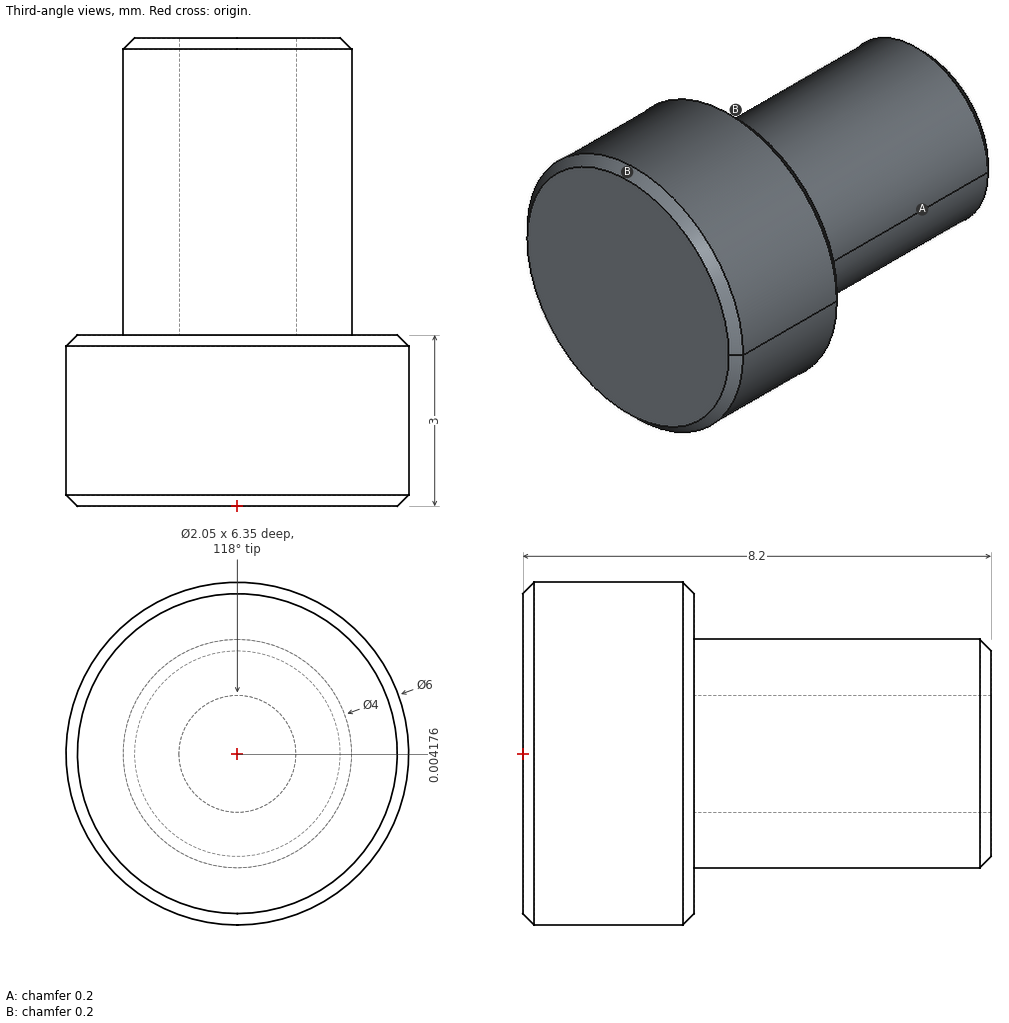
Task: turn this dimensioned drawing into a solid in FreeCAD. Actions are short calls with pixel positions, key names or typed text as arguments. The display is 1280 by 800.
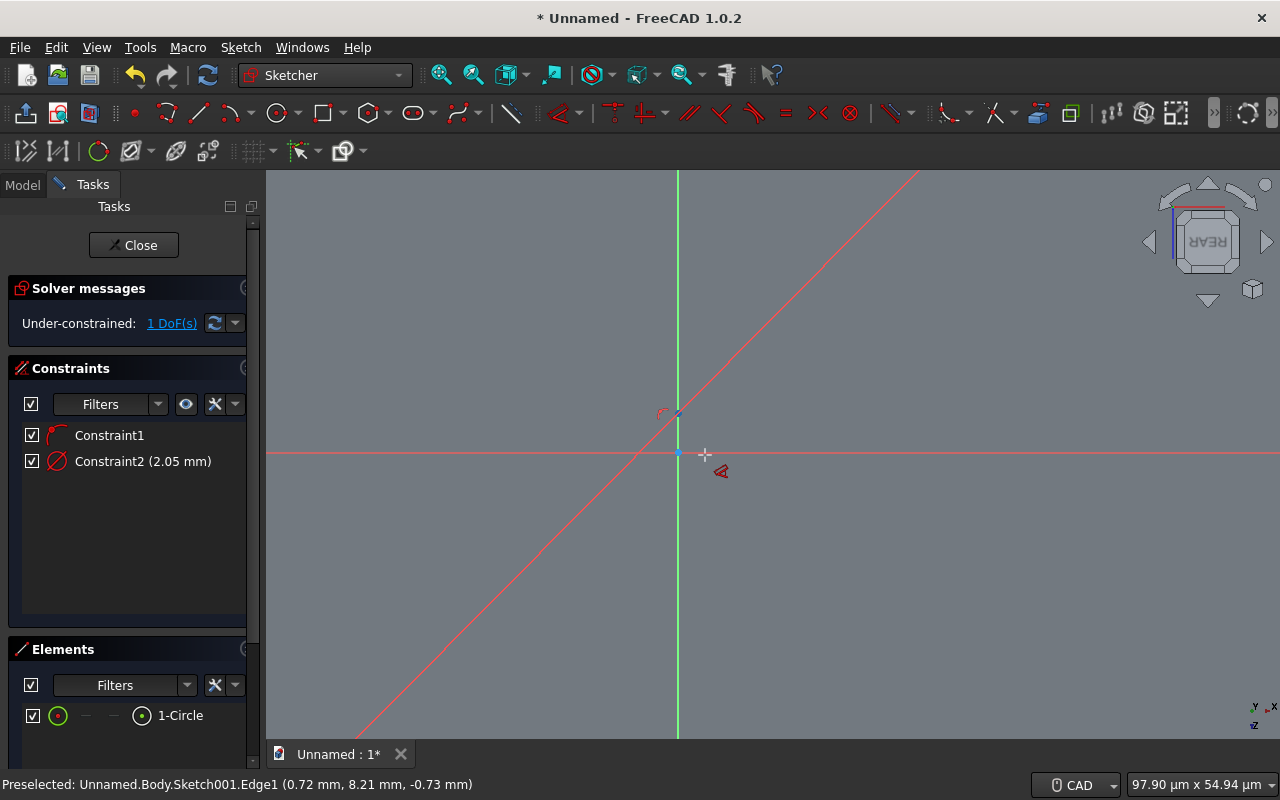
click(678, 413)
click(712, 433)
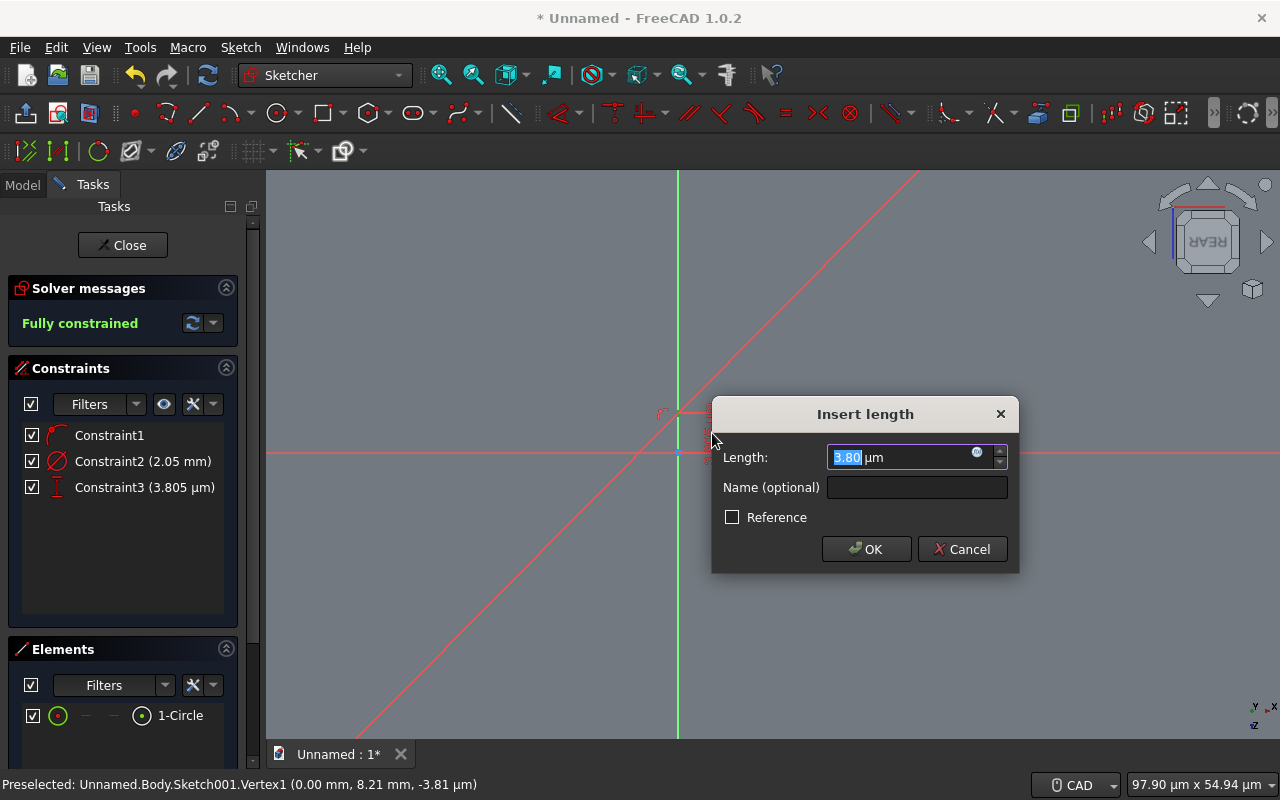
key(ctrl+a)
text(0.004176 mm)
key(Return)
key(Escape)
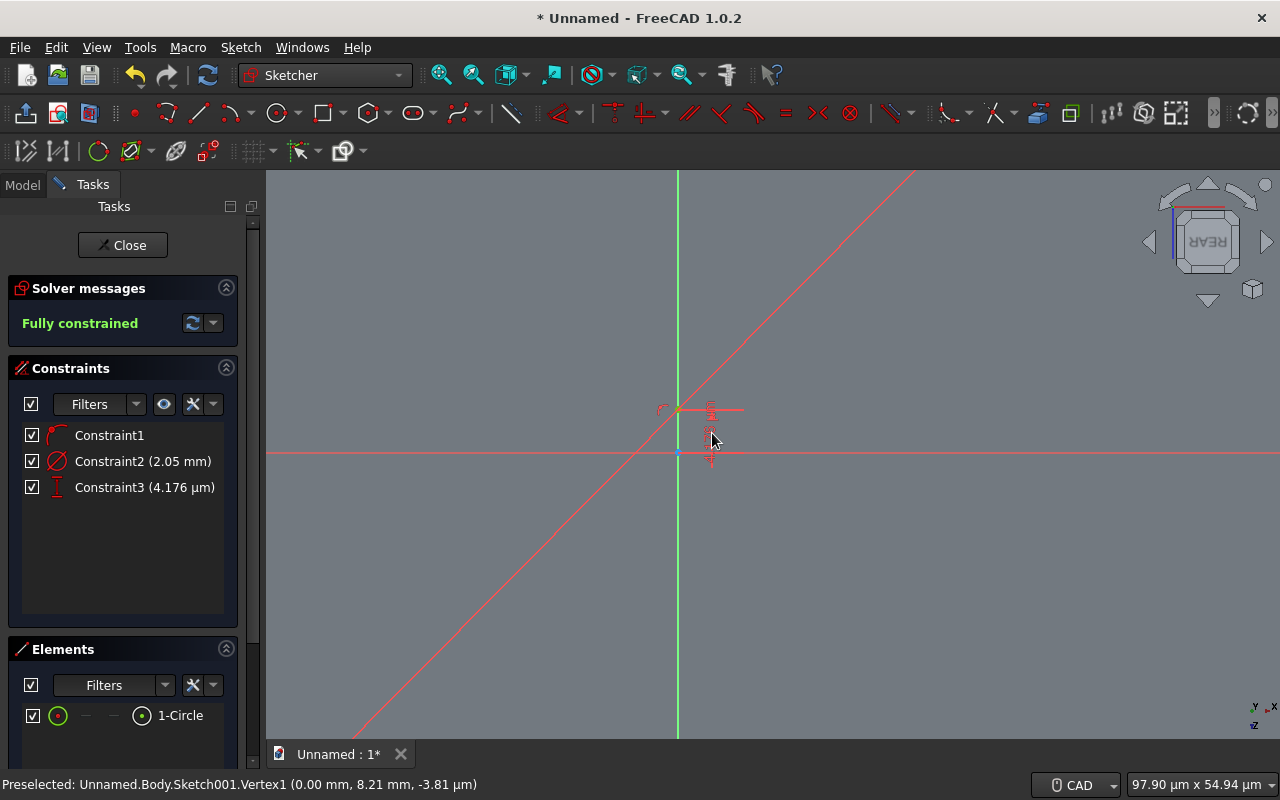
click(123, 245)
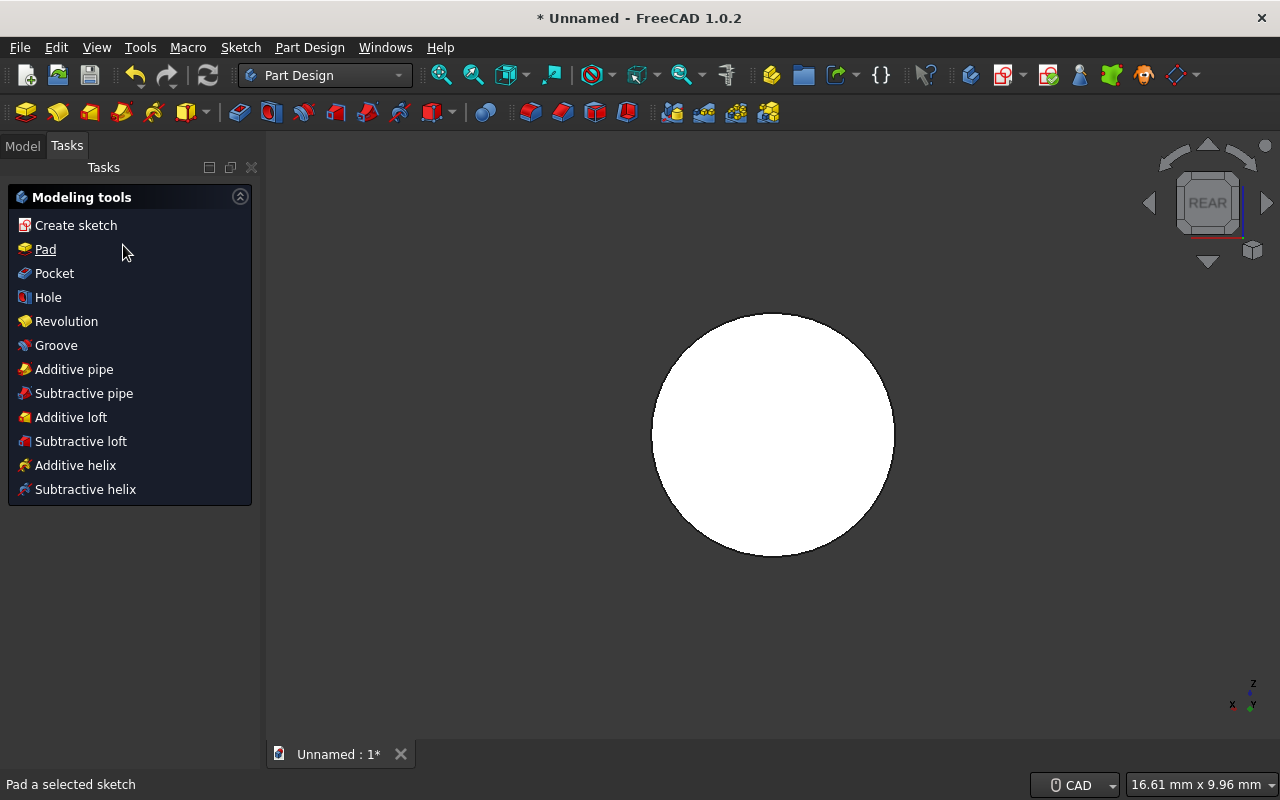
click(272, 112)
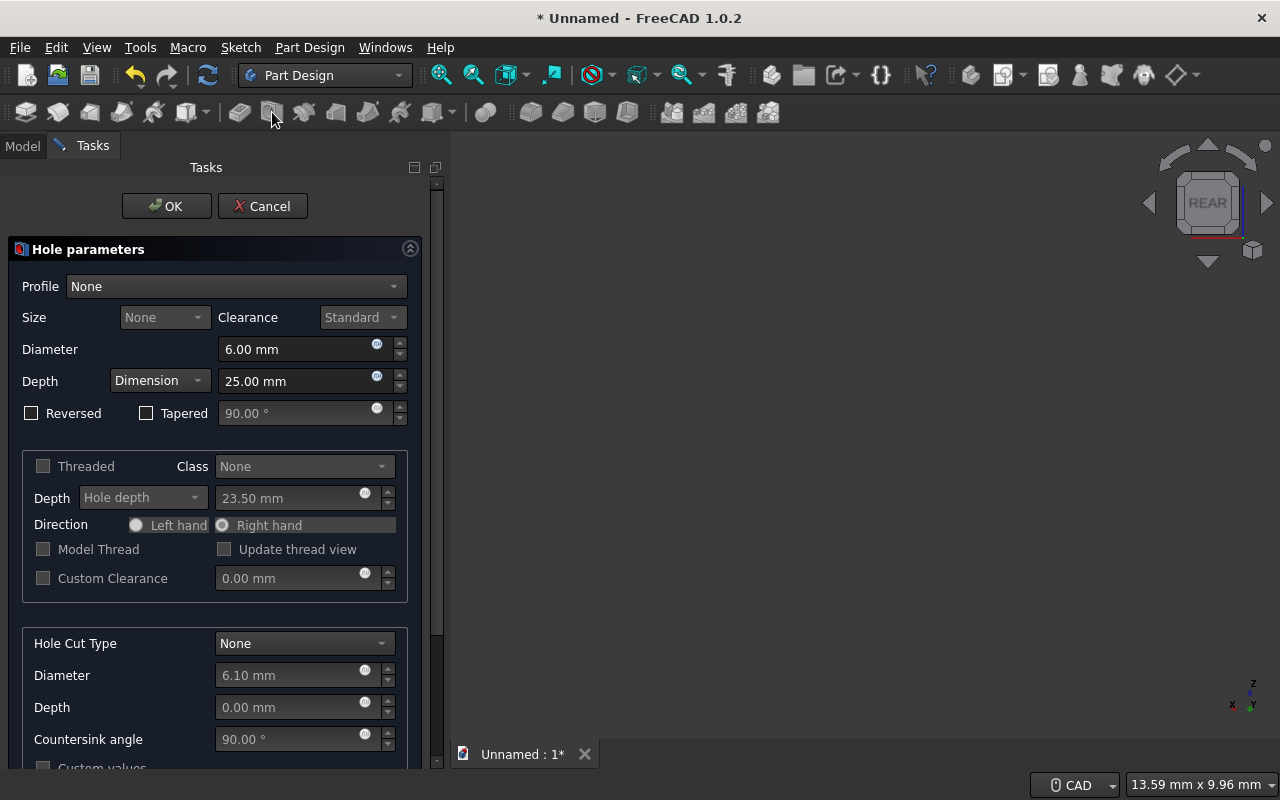
triple_click(305, 349)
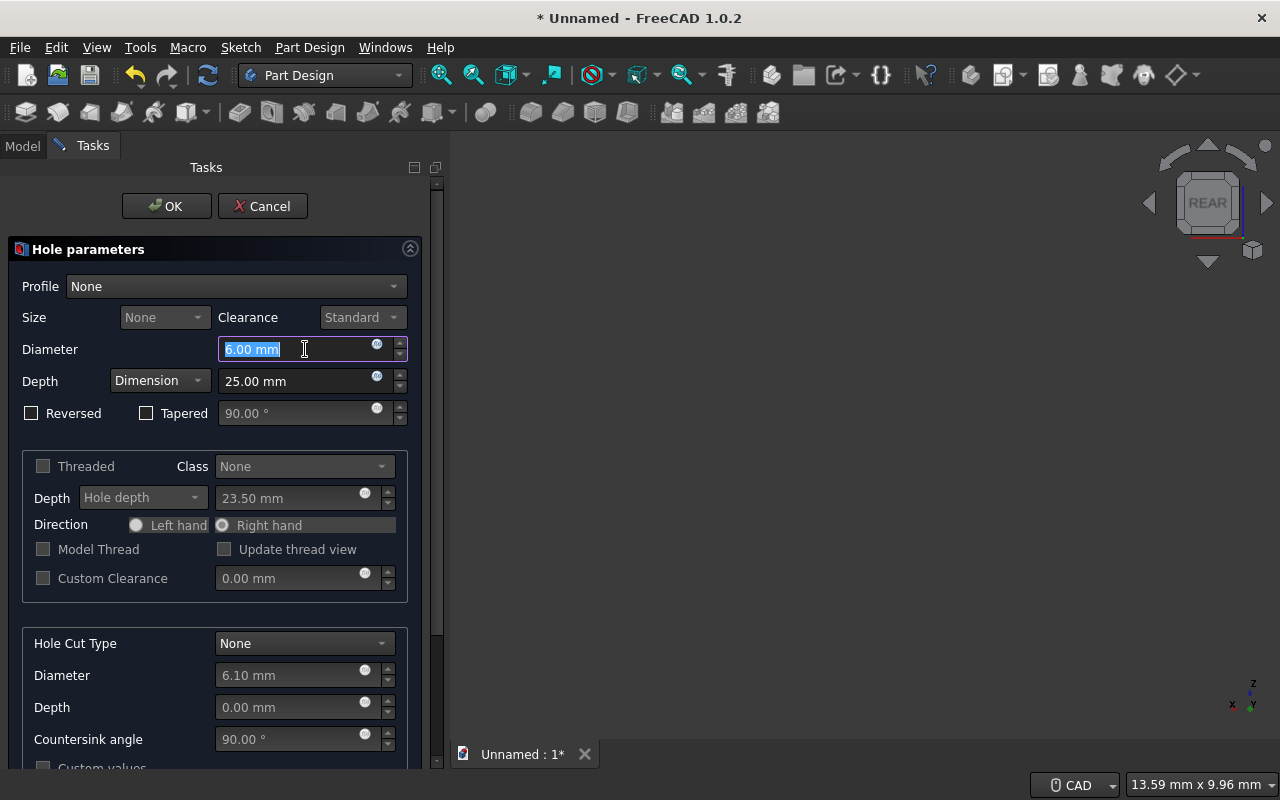
text(2.05)
key(Tab)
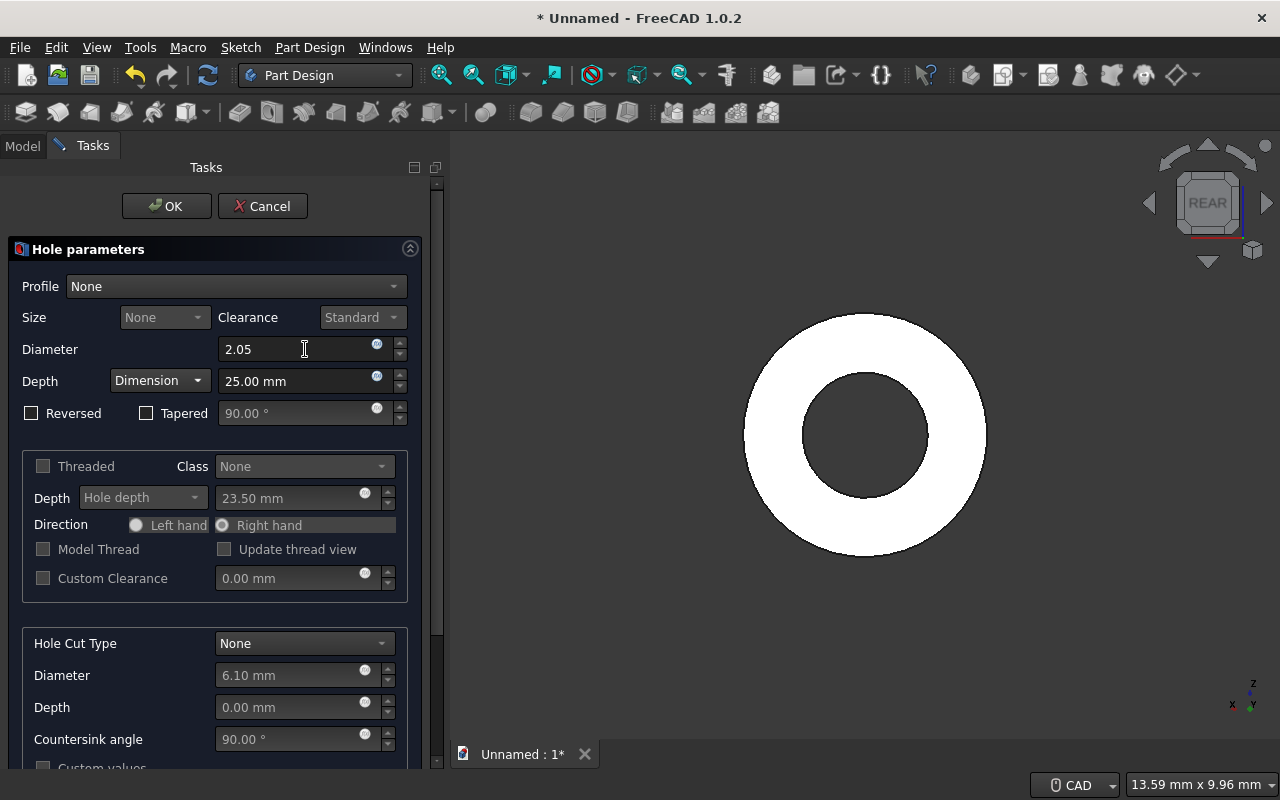
triple_click(305, 381)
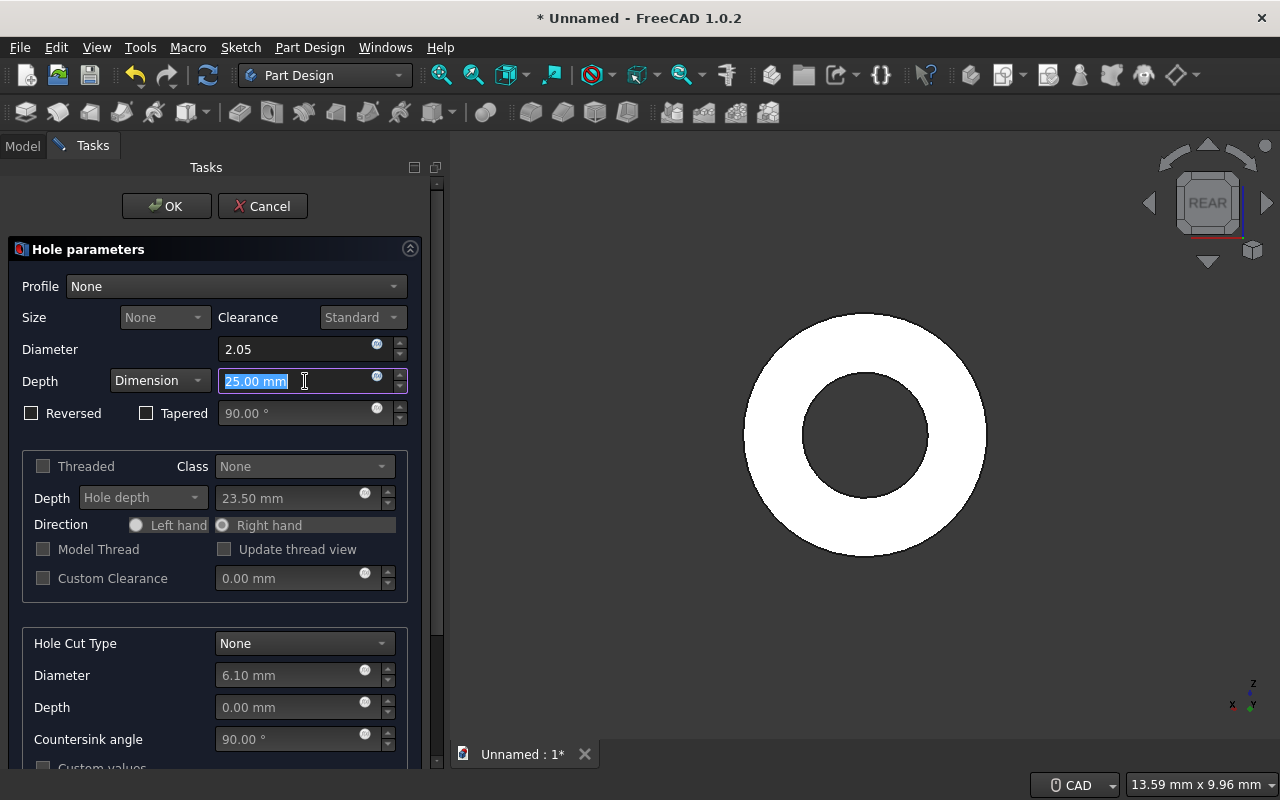
text(6.35)
key(Tab)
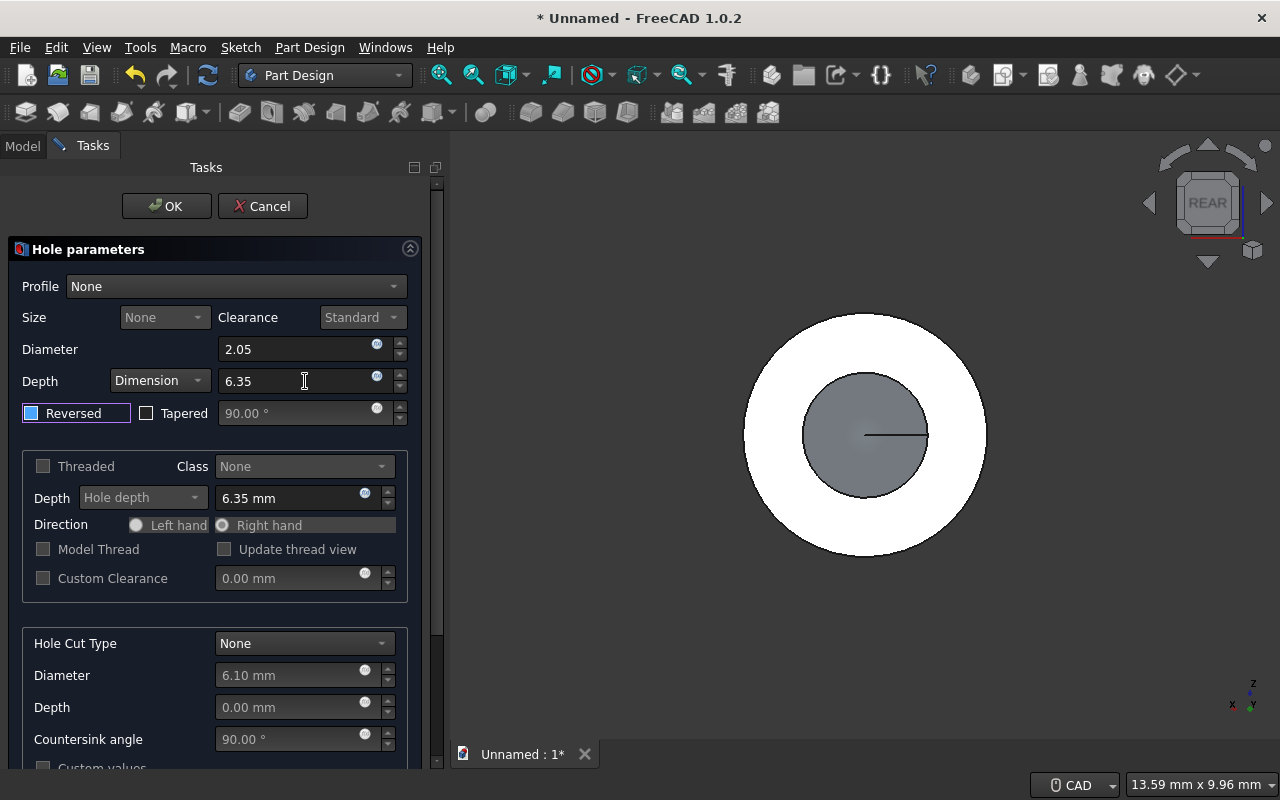
click(167, 206)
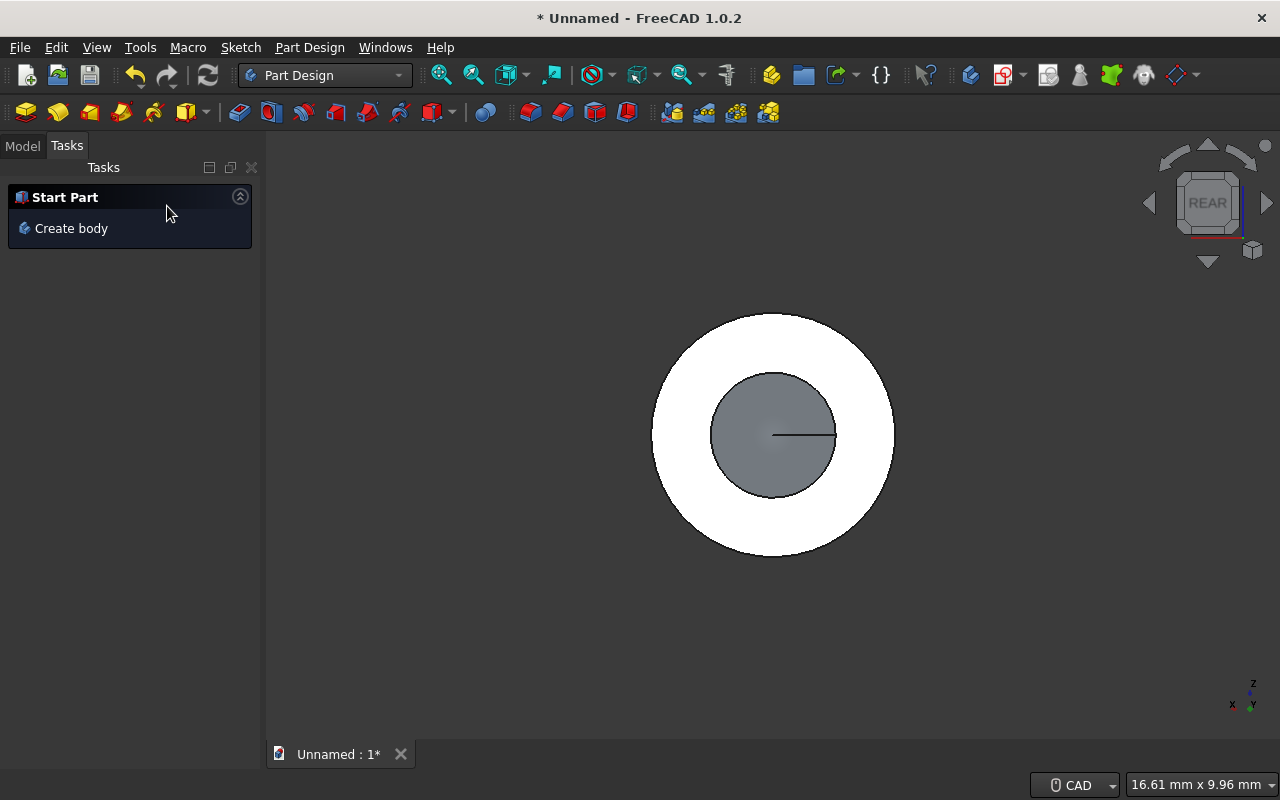
click(442, 76)